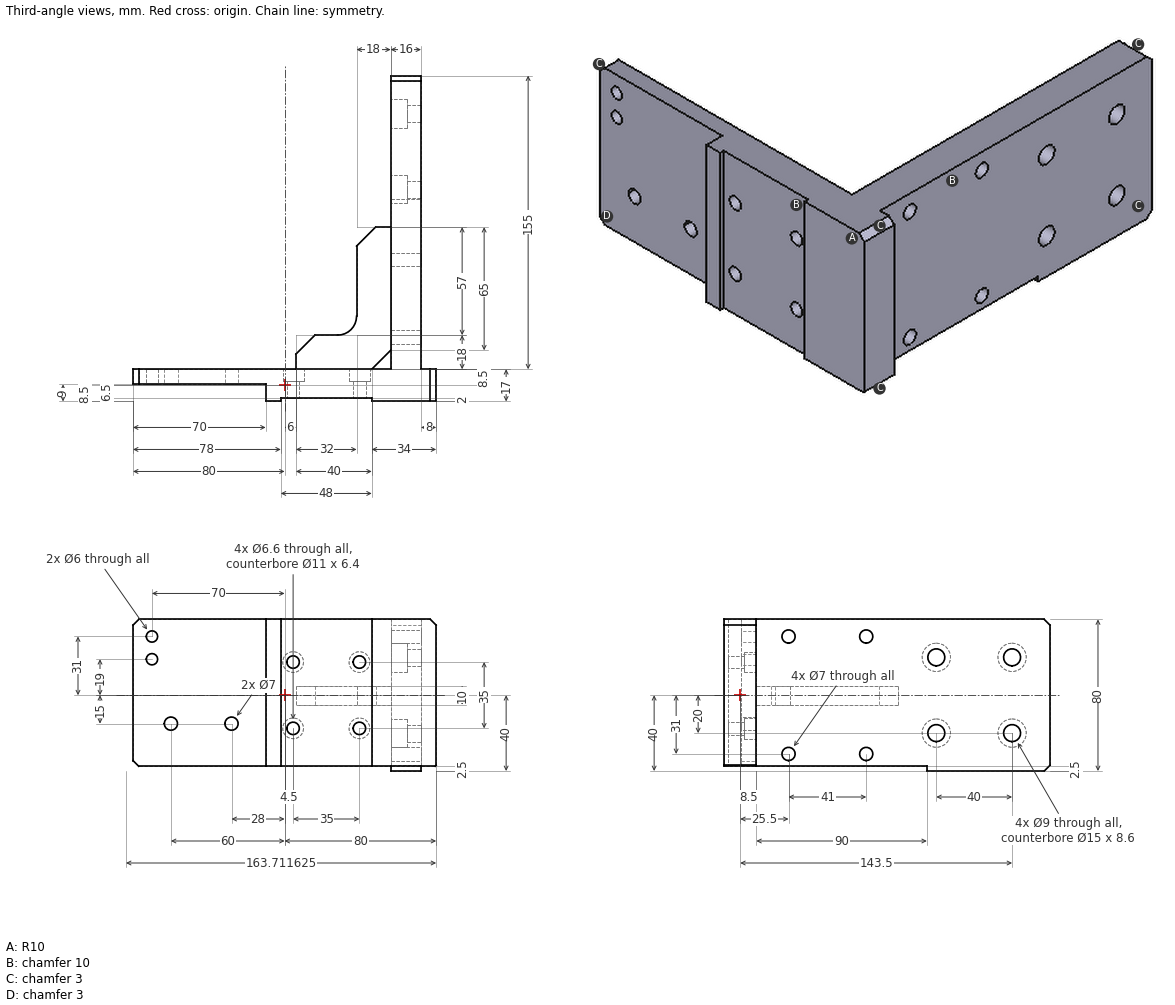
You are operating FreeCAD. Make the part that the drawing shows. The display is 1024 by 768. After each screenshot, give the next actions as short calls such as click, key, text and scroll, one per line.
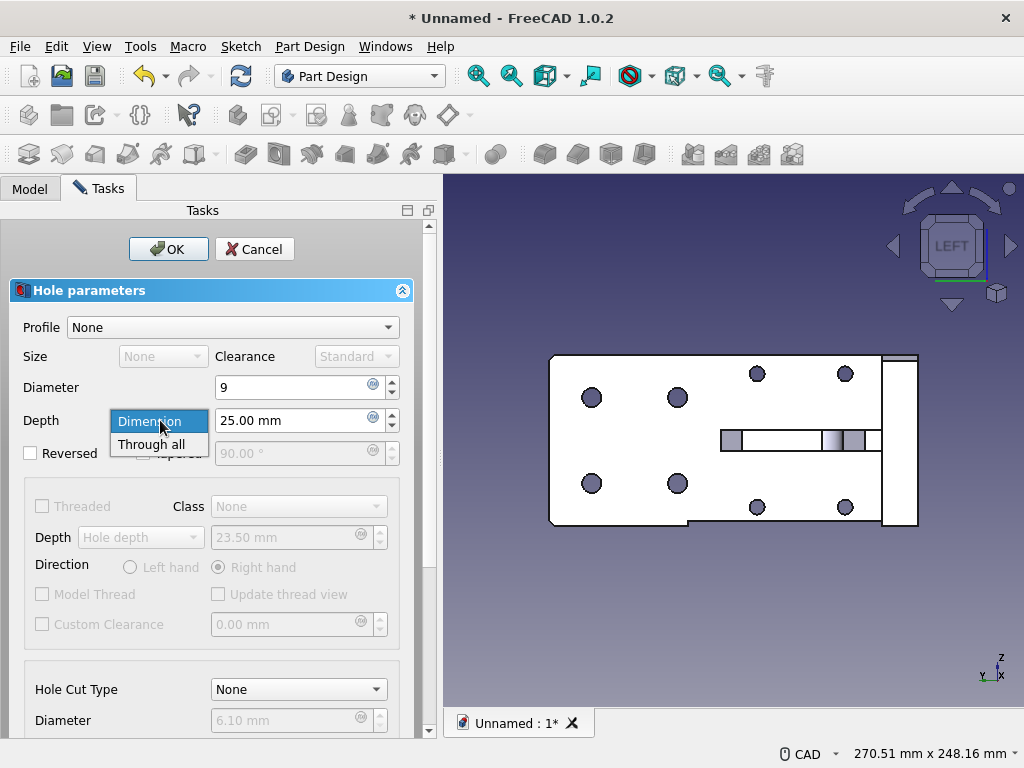
click(158, 444)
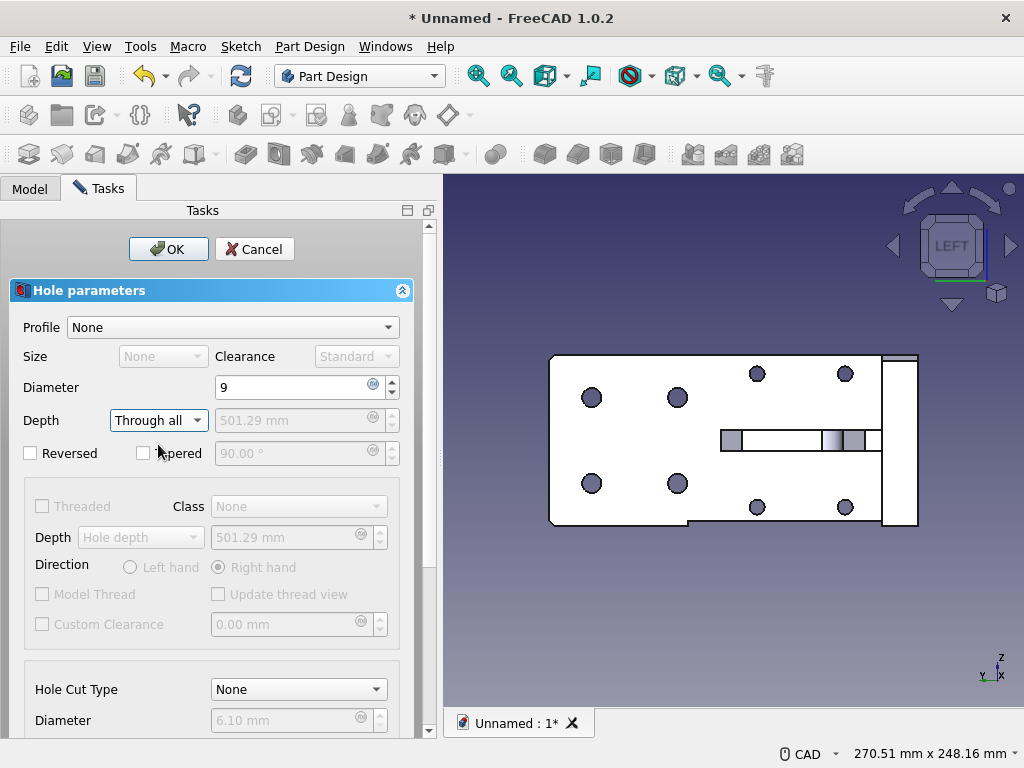
click(300, 690)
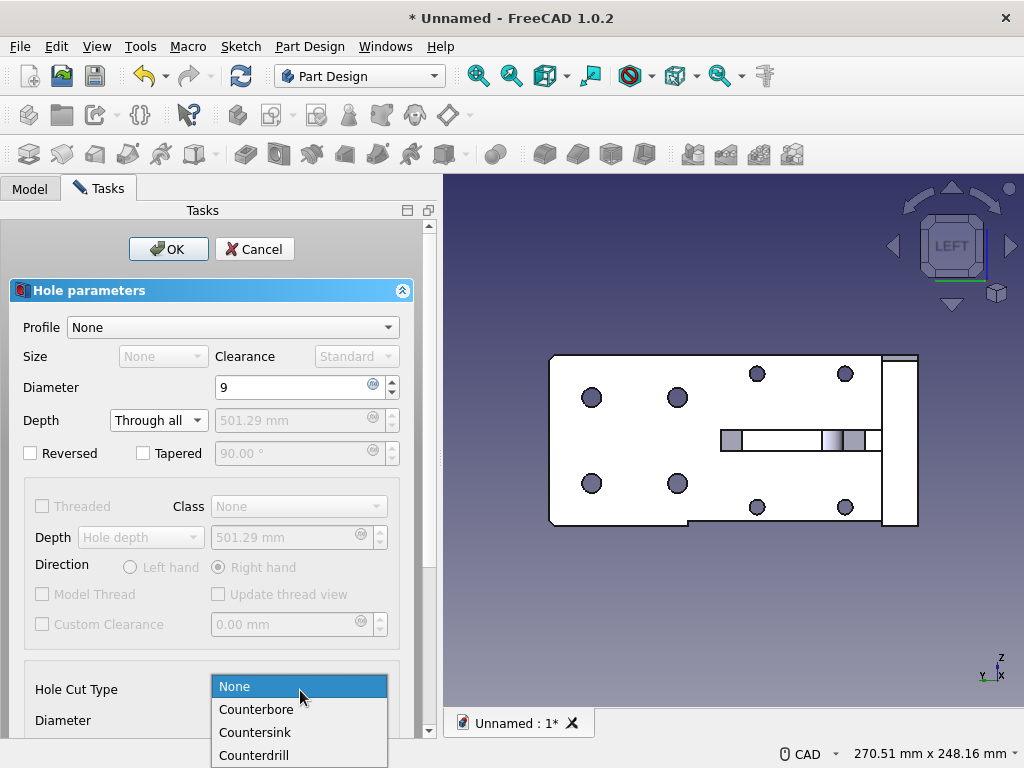
click(298, 710)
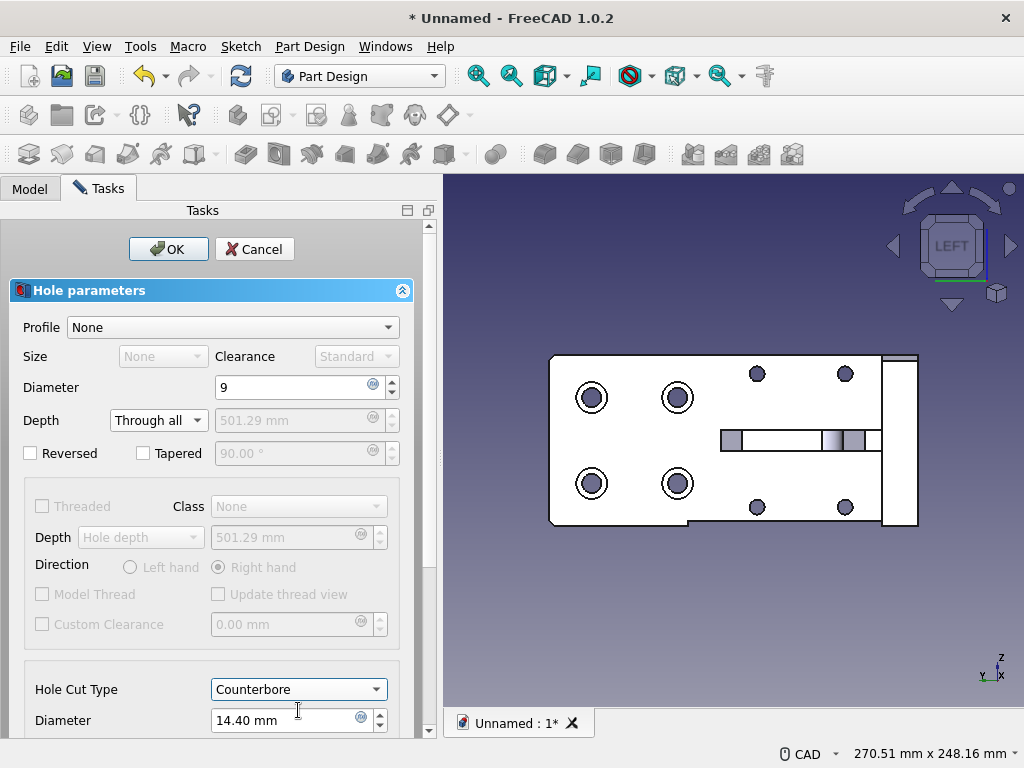
triple_click(292, 720)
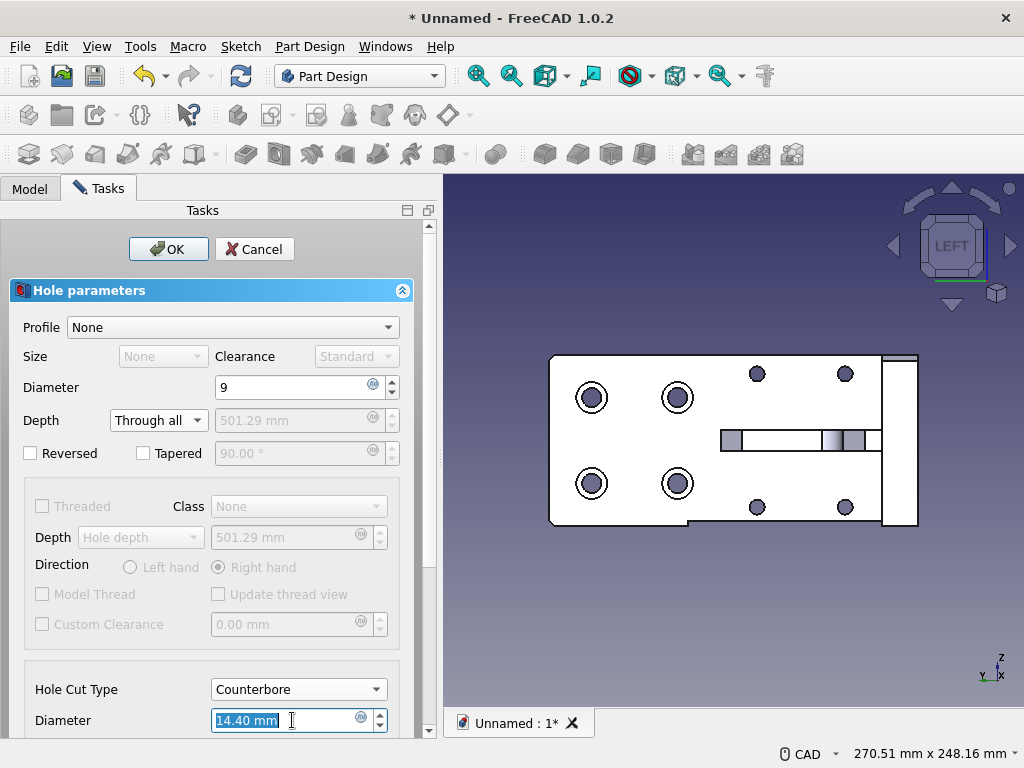
text(15)
key(Tab)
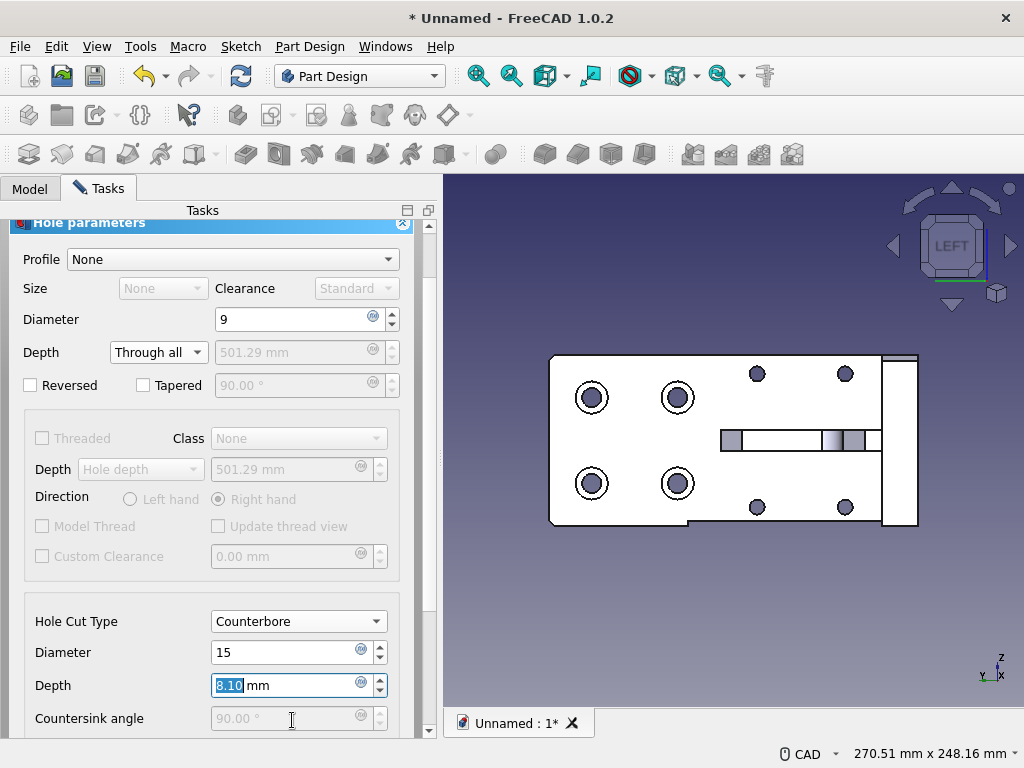
text(8.6)
key(Tab)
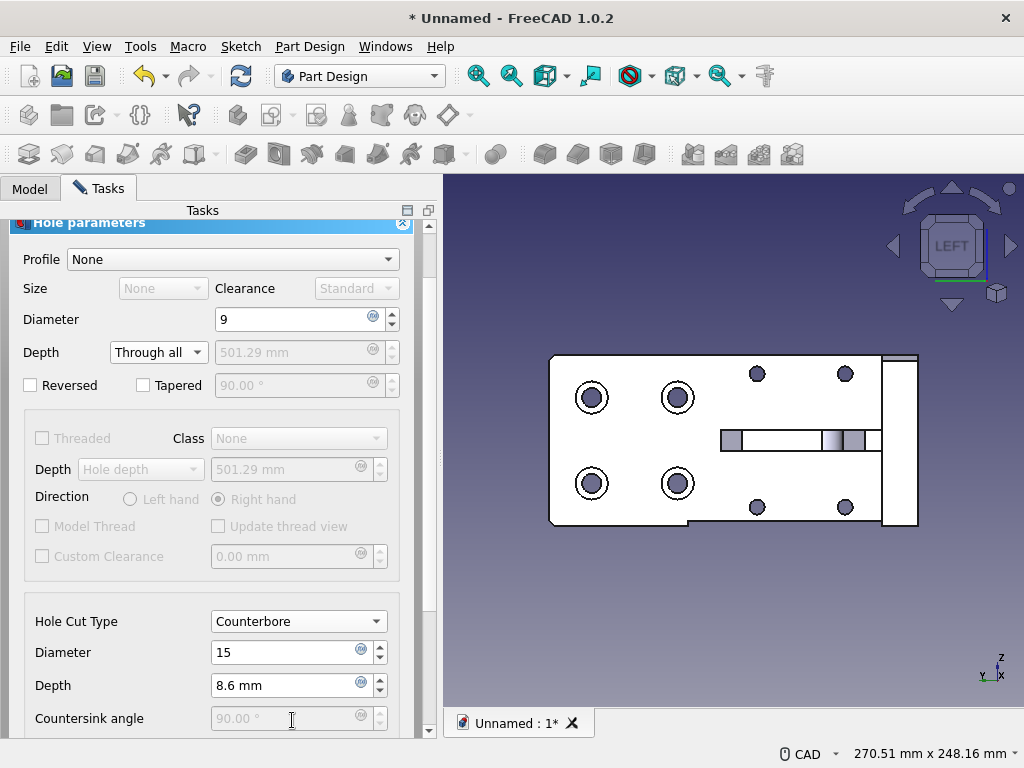
scroll(429, 479, up, 2)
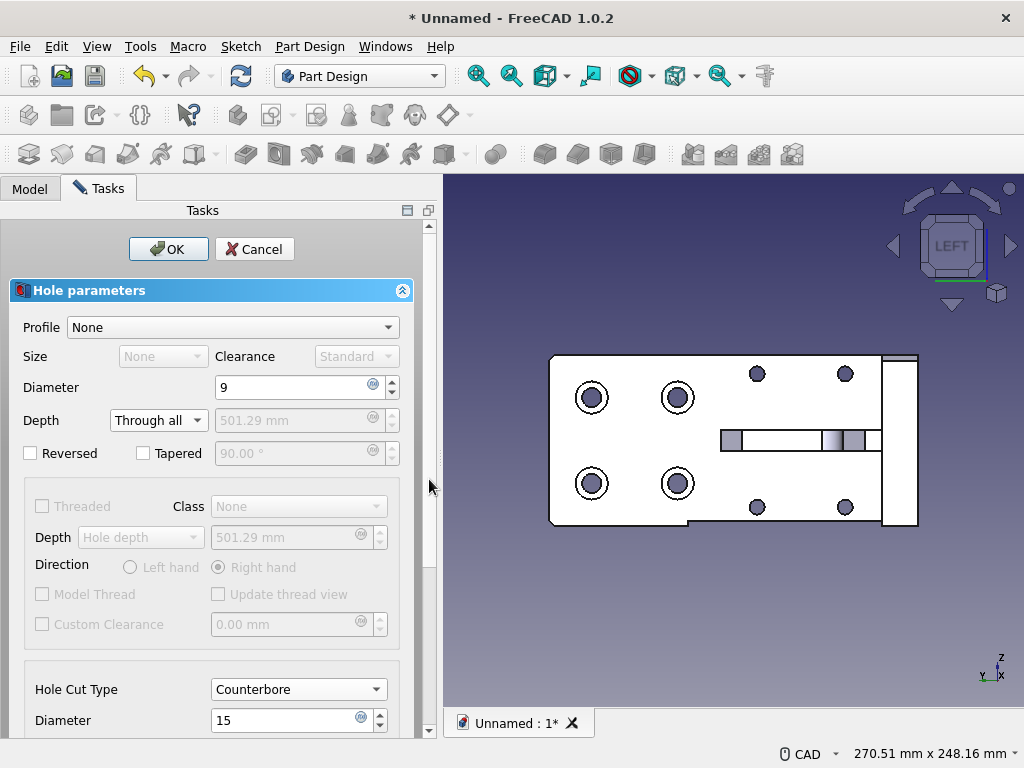
click(169, 249)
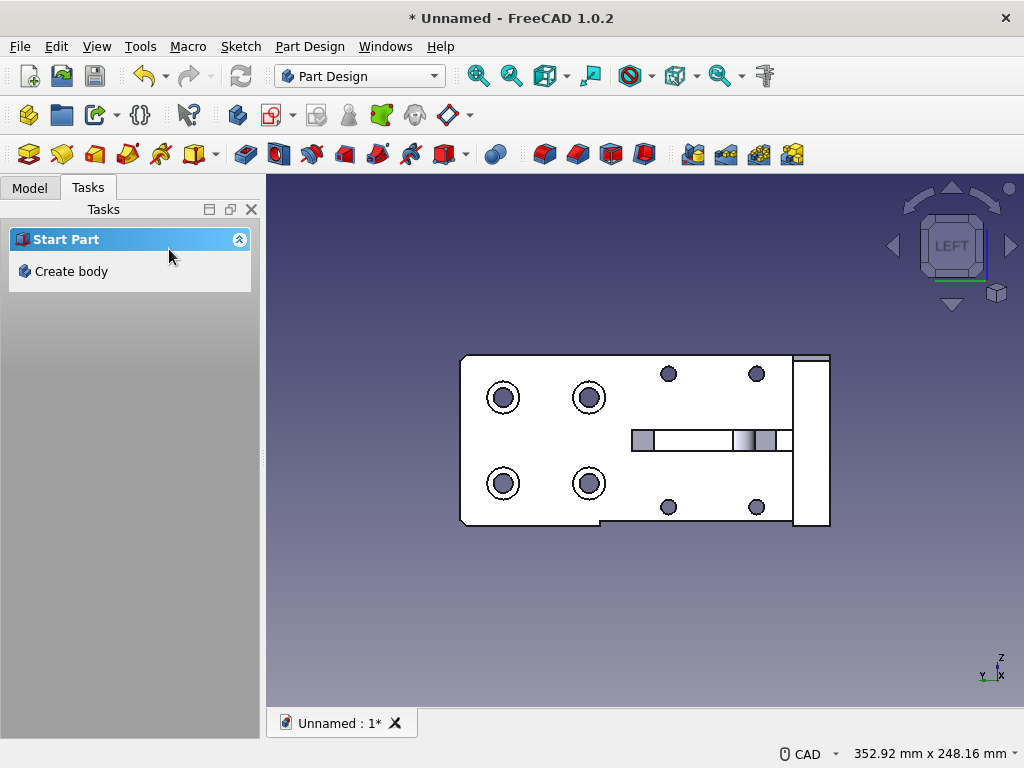
key(4)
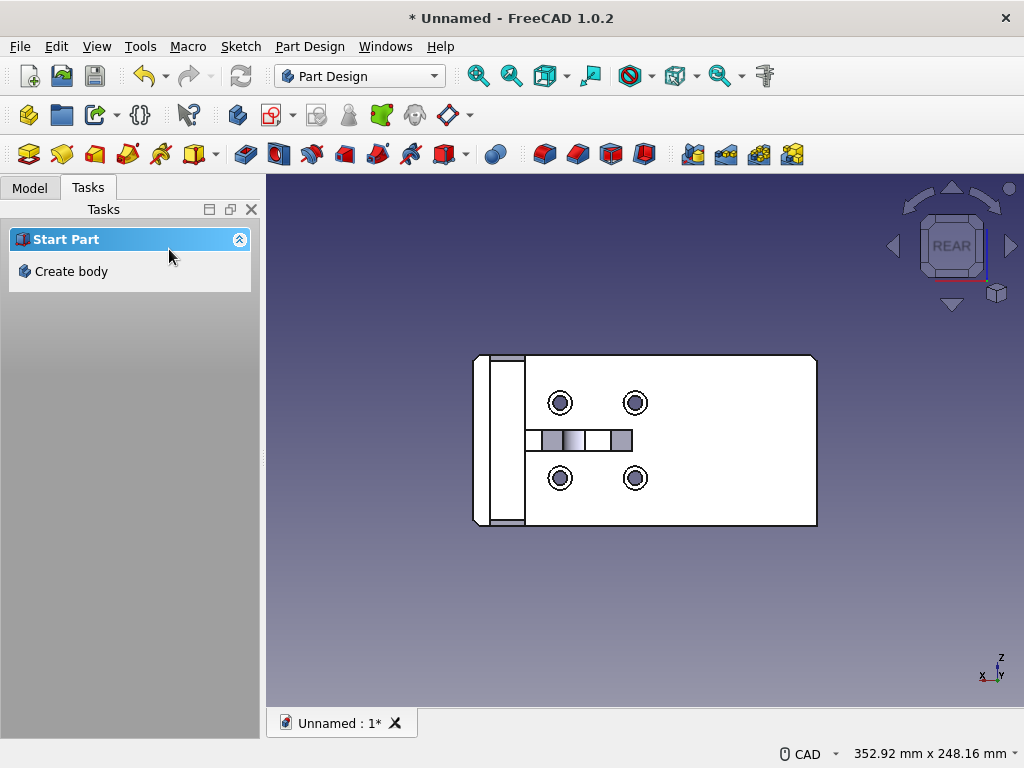
click(743, 440)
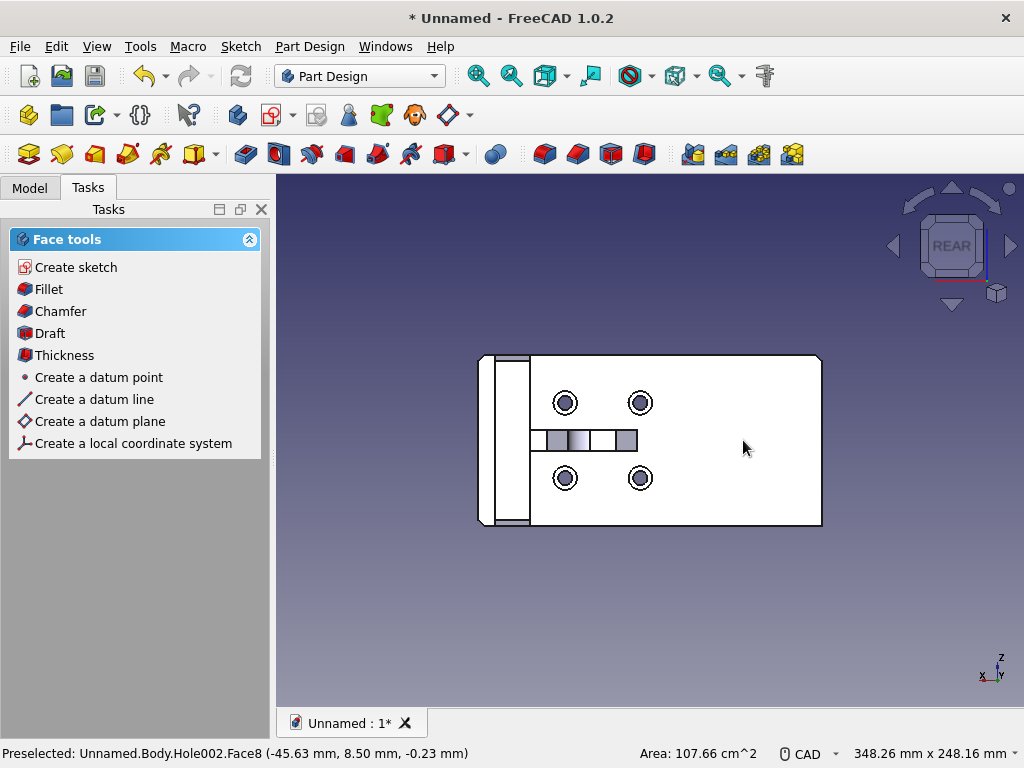
click(270, 116)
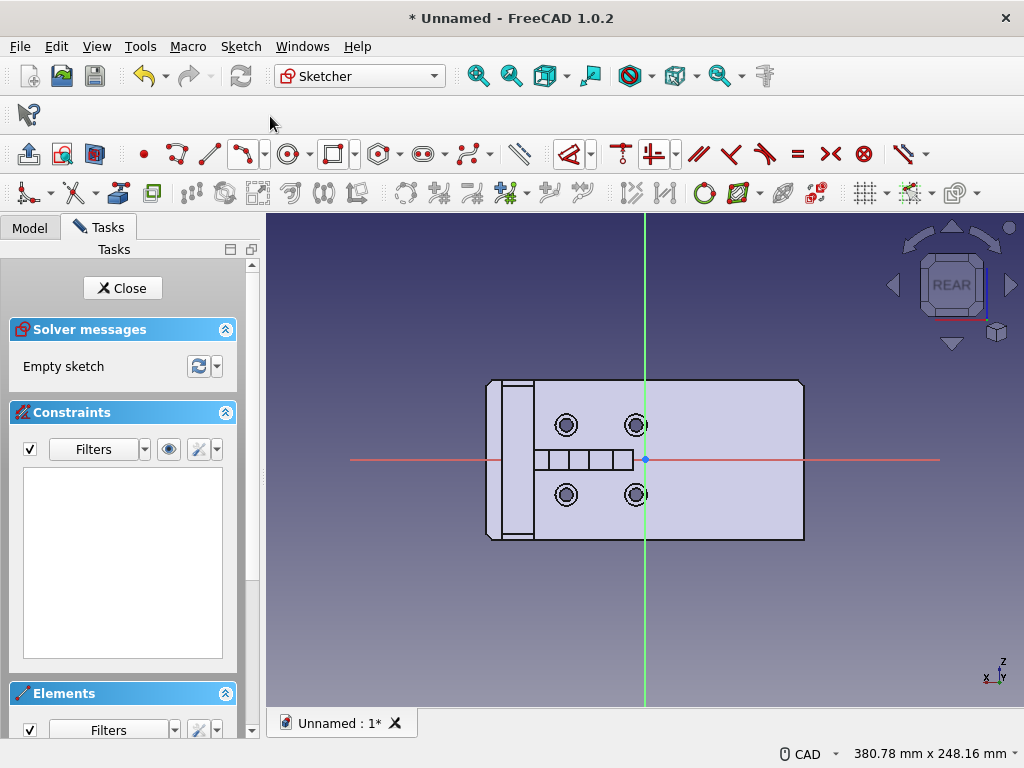
click(95, 154)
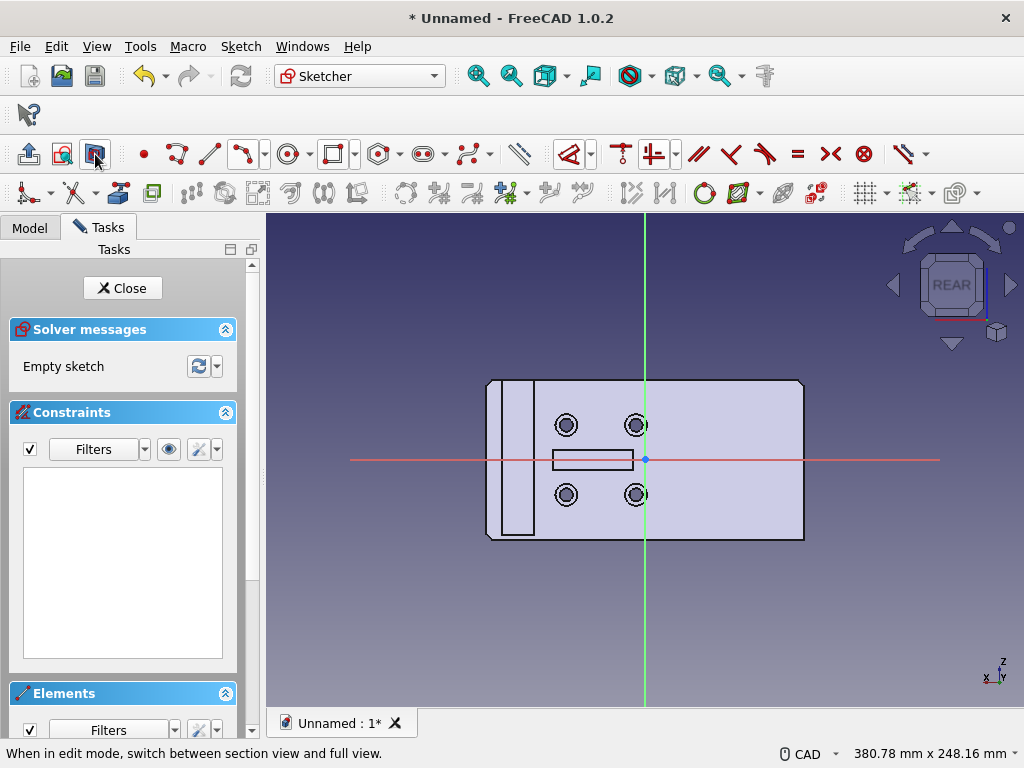
key(g)
key(r)